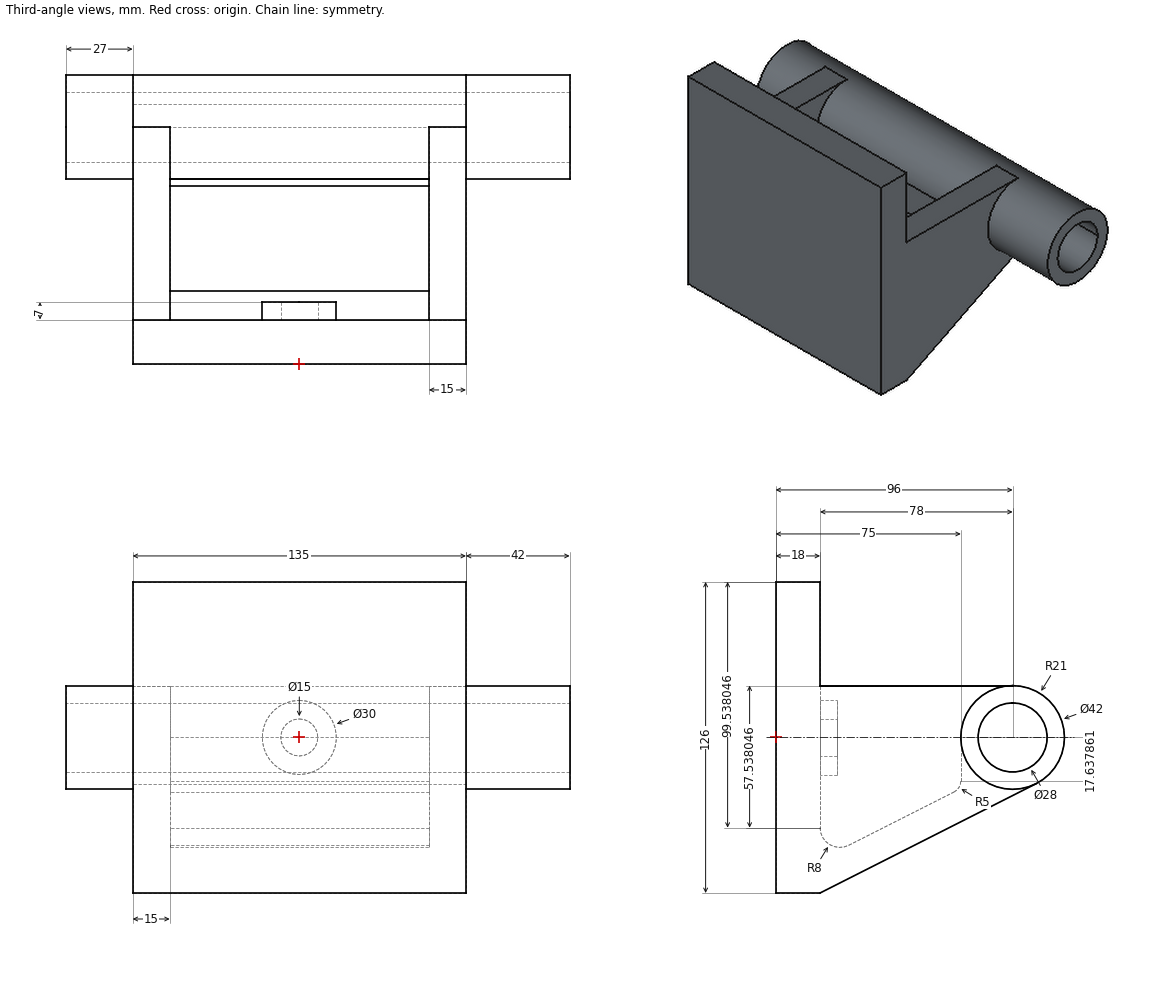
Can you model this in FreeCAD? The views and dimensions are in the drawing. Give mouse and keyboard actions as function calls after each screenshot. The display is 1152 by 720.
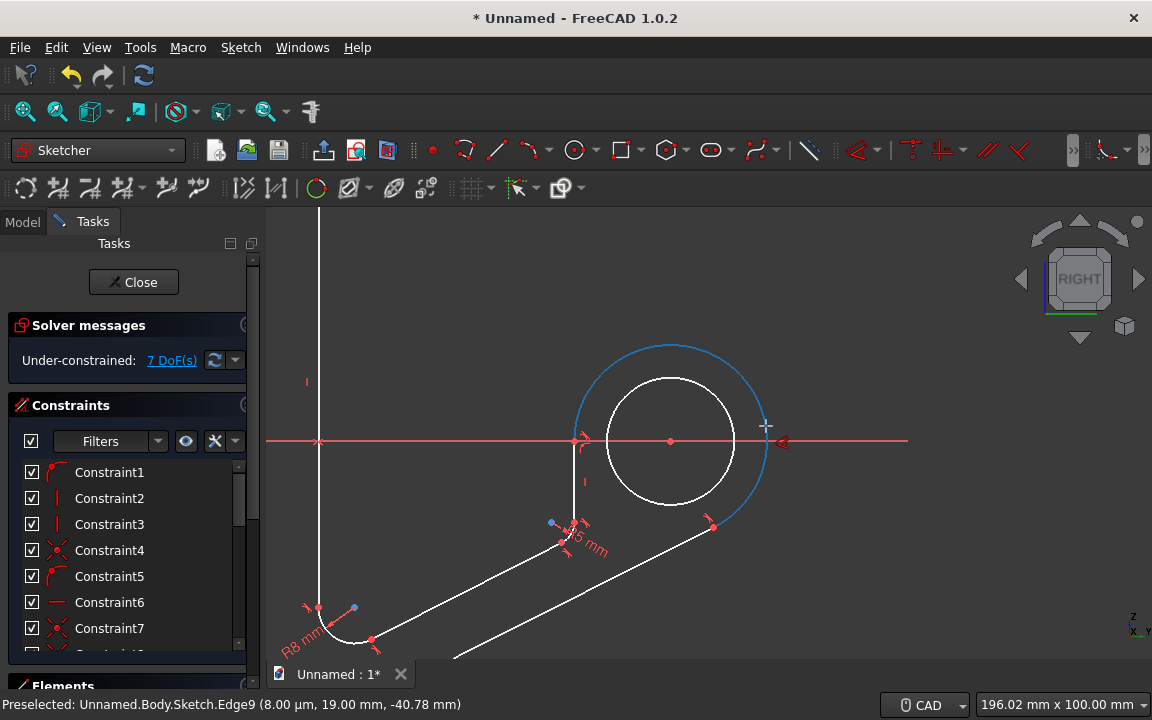
click(765, 425)
click(797, 420)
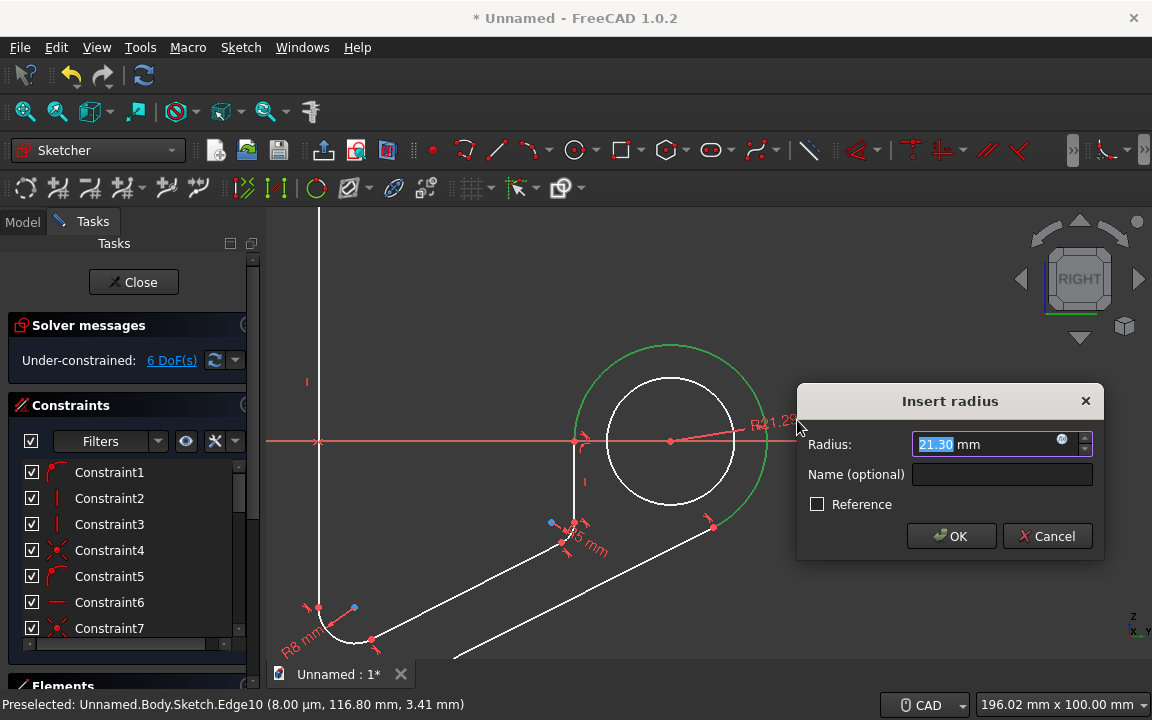
text(21)
key(Return)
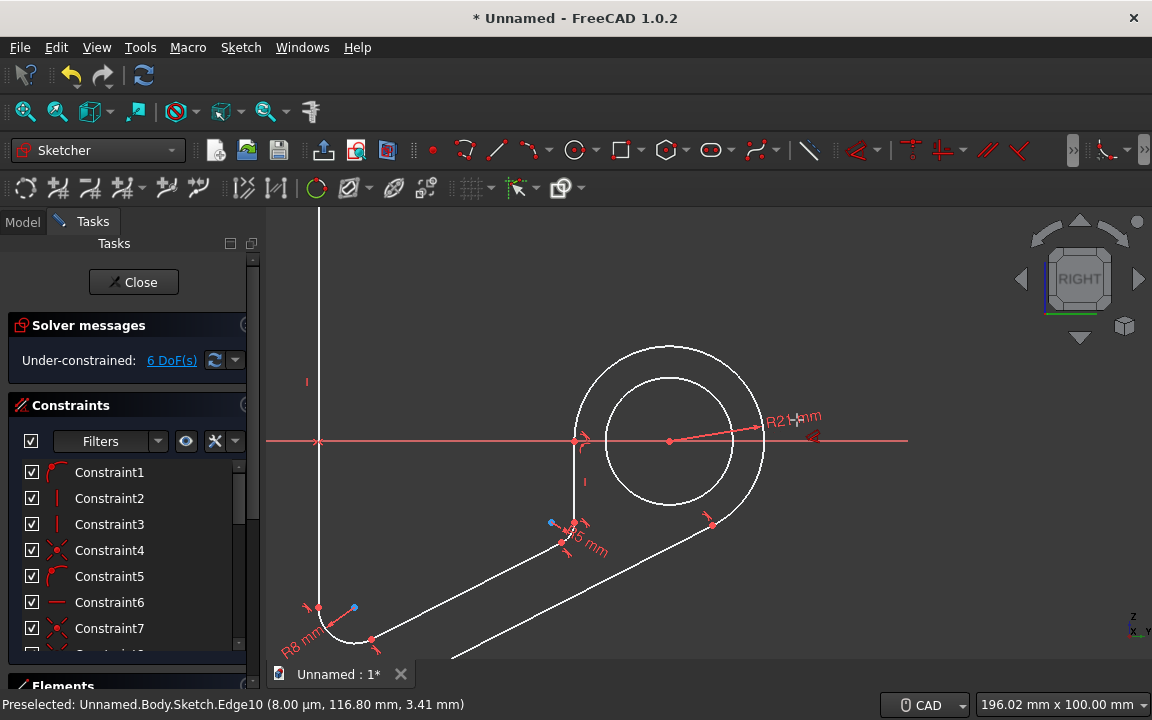
click(714, 396)
click(602, 510)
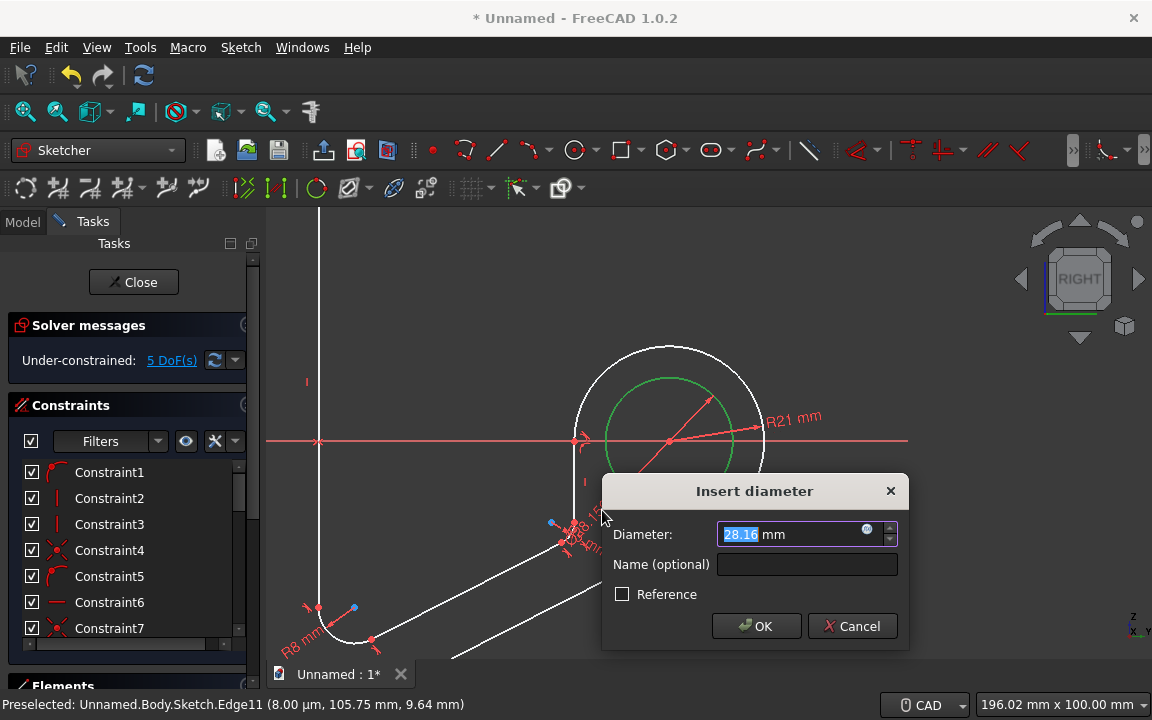
text(28)
key(Return)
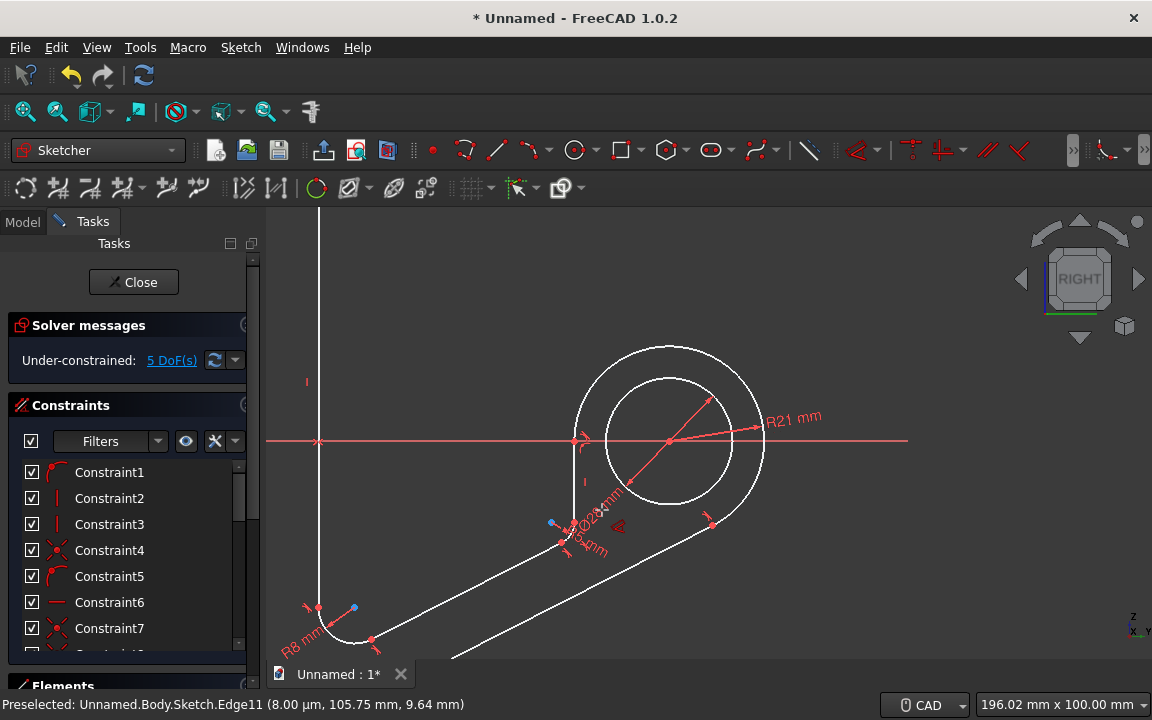
scroll(766, 426, down, 4)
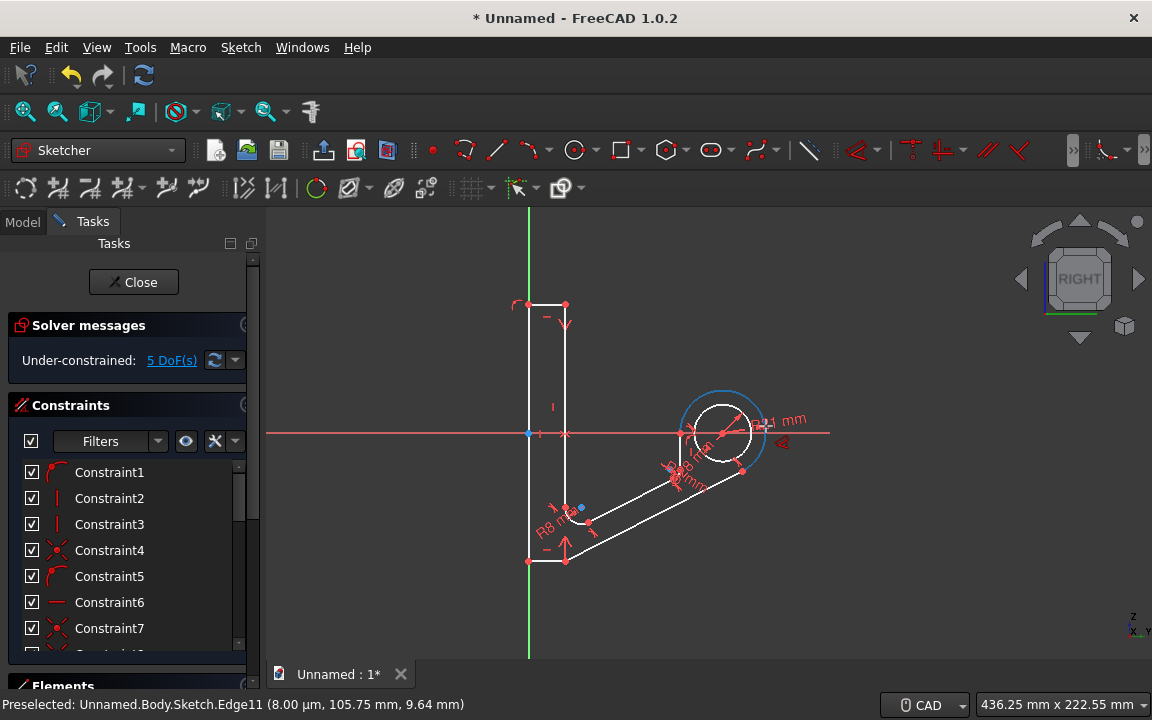
scroll(554, 305, up, 2)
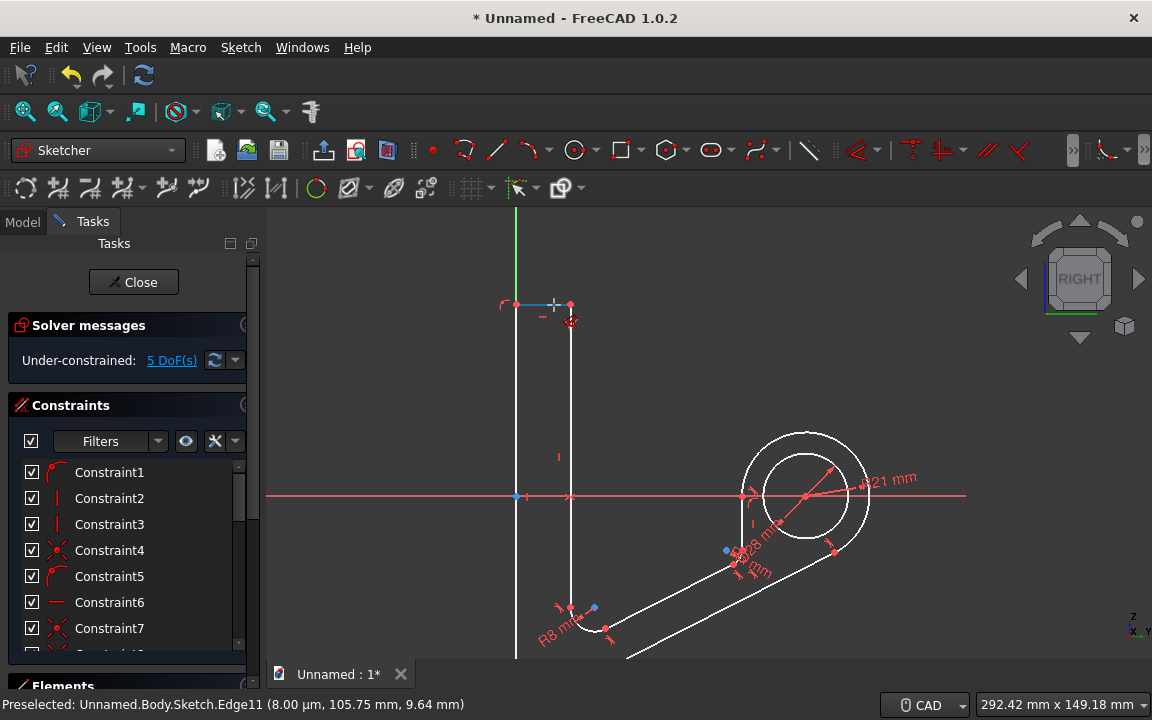
click(554, 305)
click(544, 271)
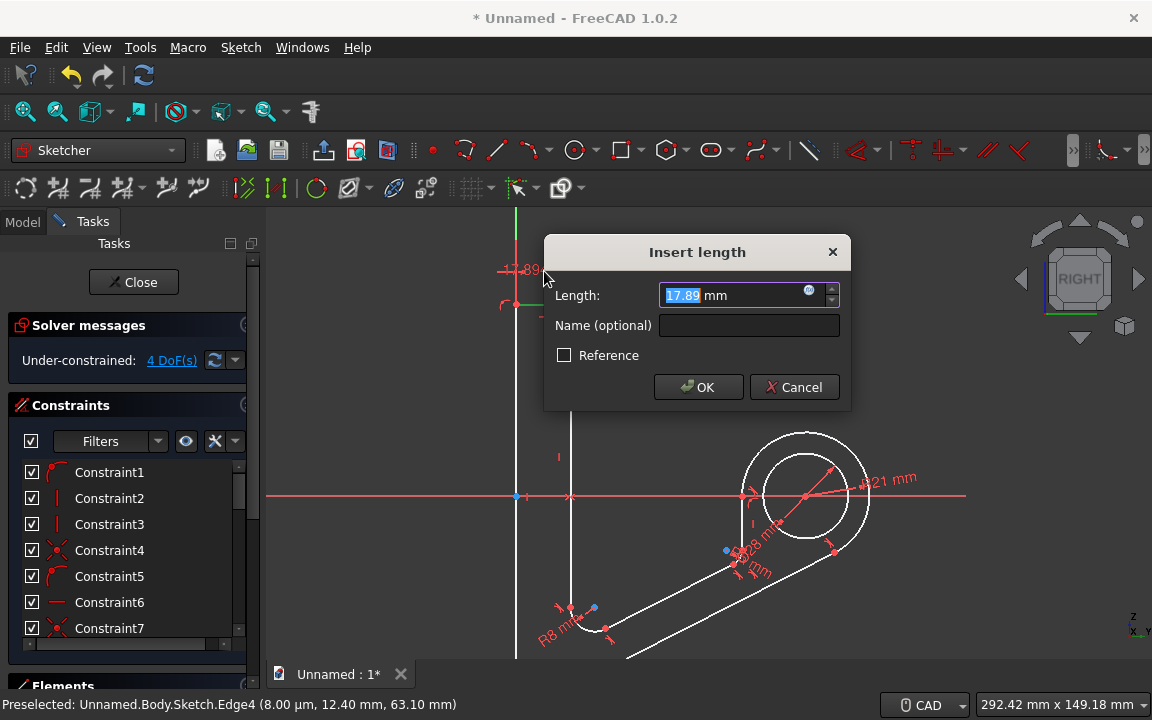
text(18)
key(Return)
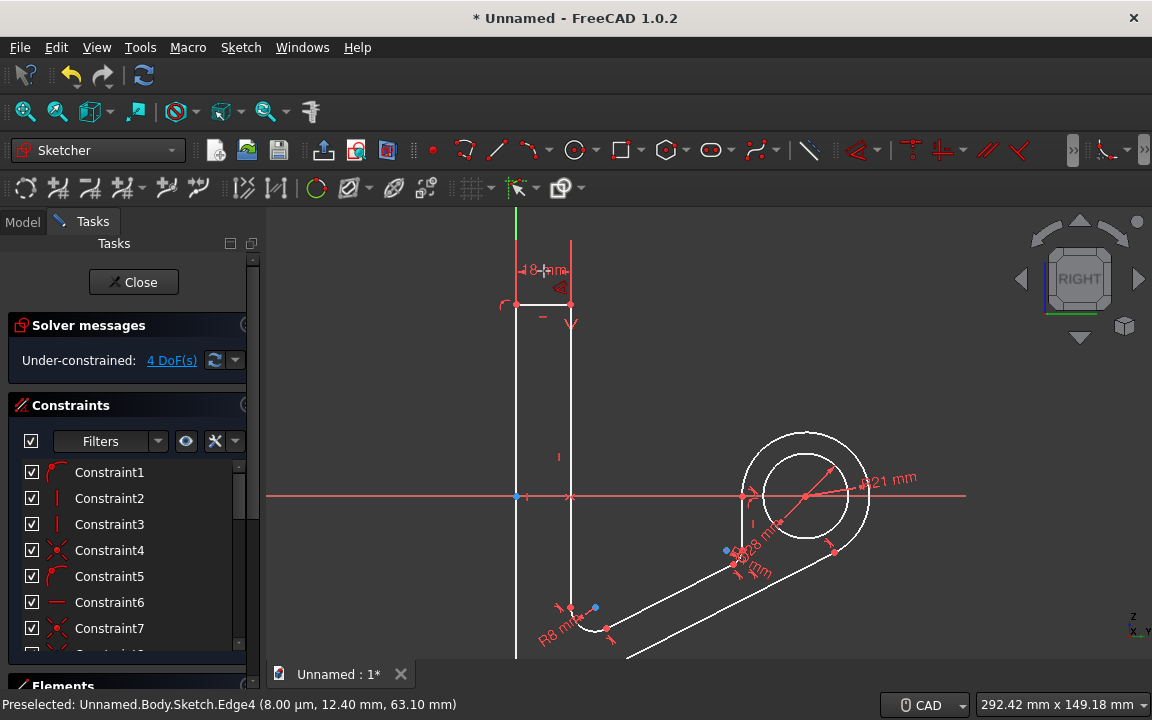
click(806, 496)
click(661, 530)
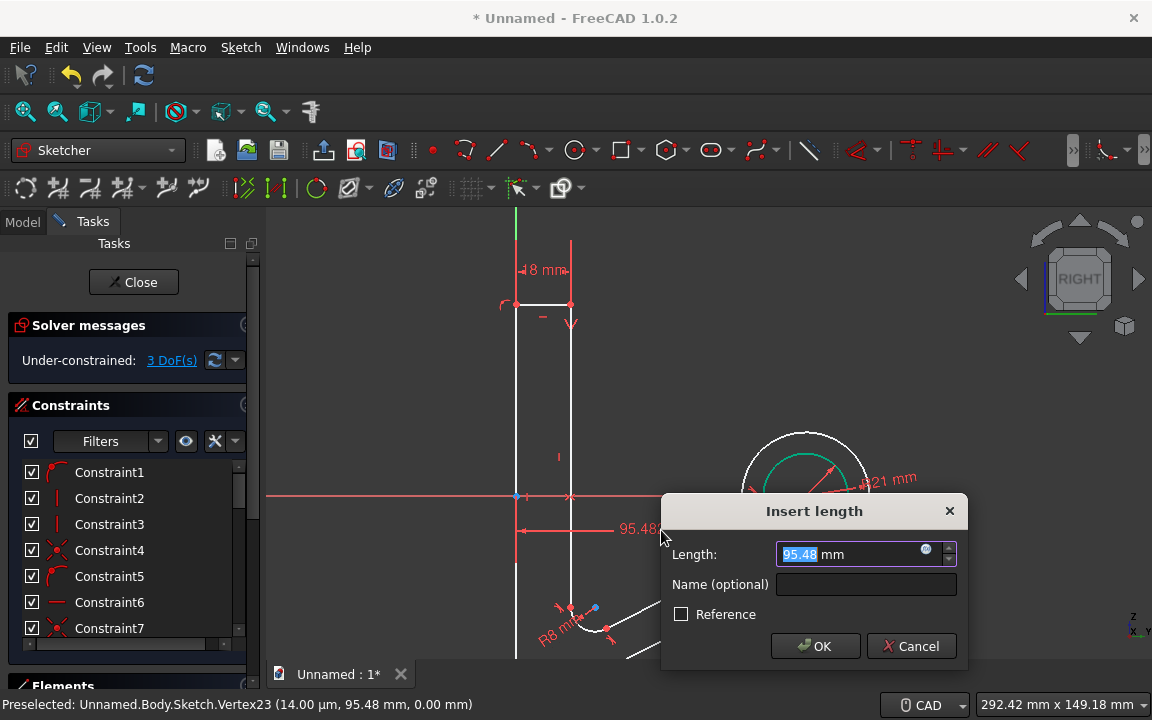
text(96)
key(Return)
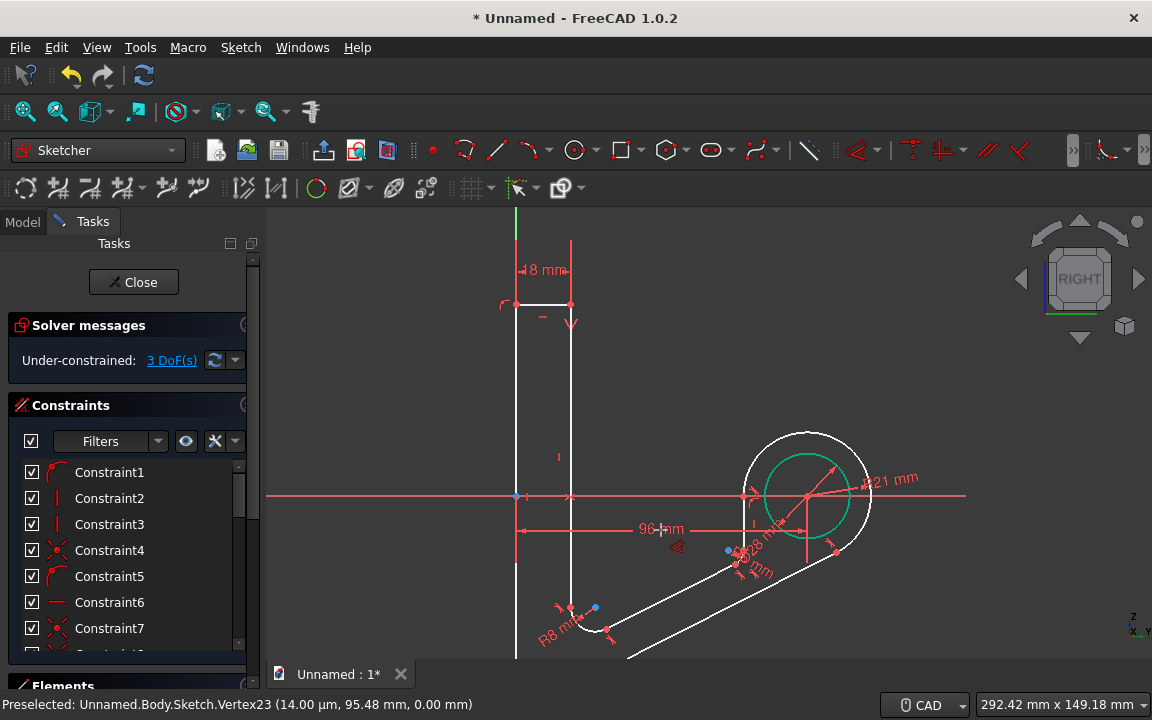
click(516, 420)
click(482, 468)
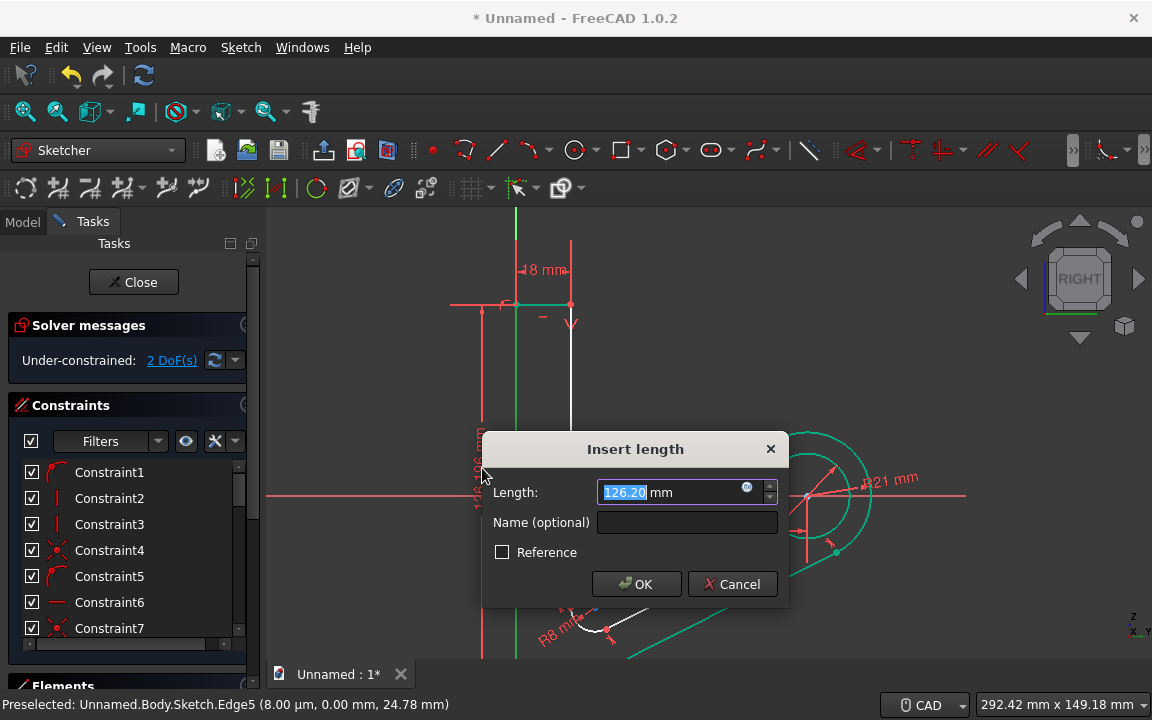
text(126)
key(Return)